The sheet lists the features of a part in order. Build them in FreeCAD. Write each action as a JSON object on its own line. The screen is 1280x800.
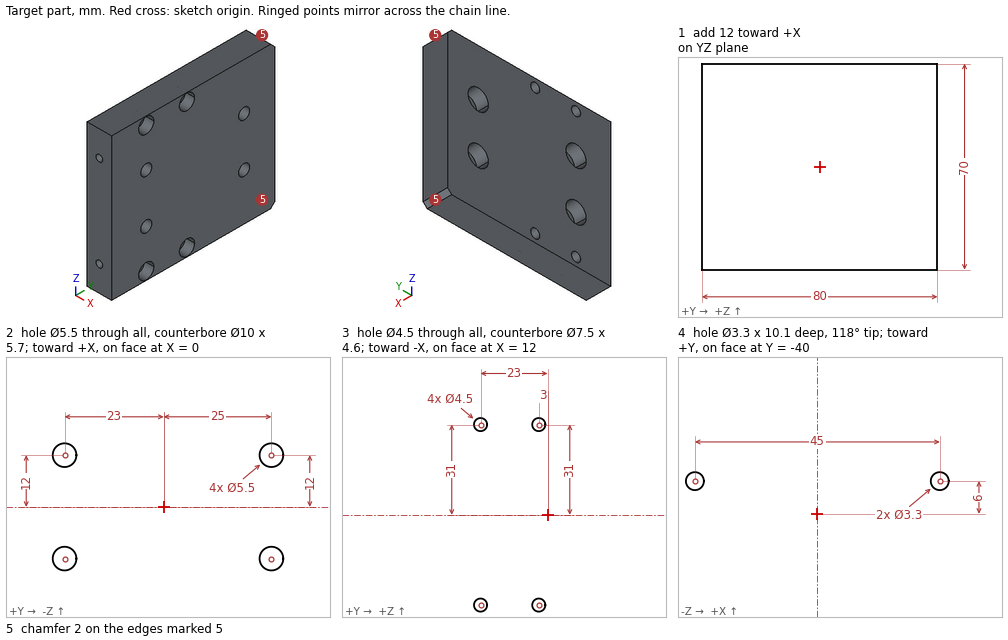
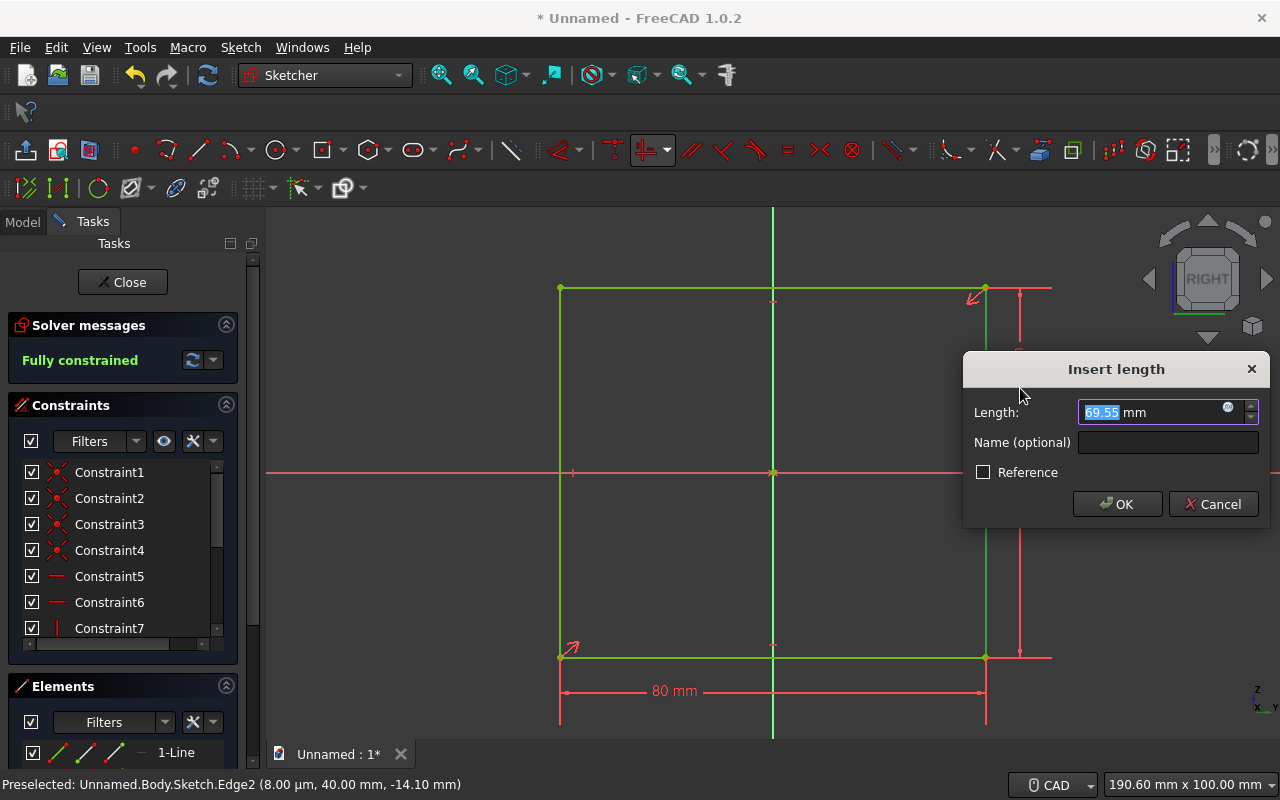
{"action": "type", "text": "70"}
{"action": "key", "text": "Return"}
{"action": "key", "text": "Escape"}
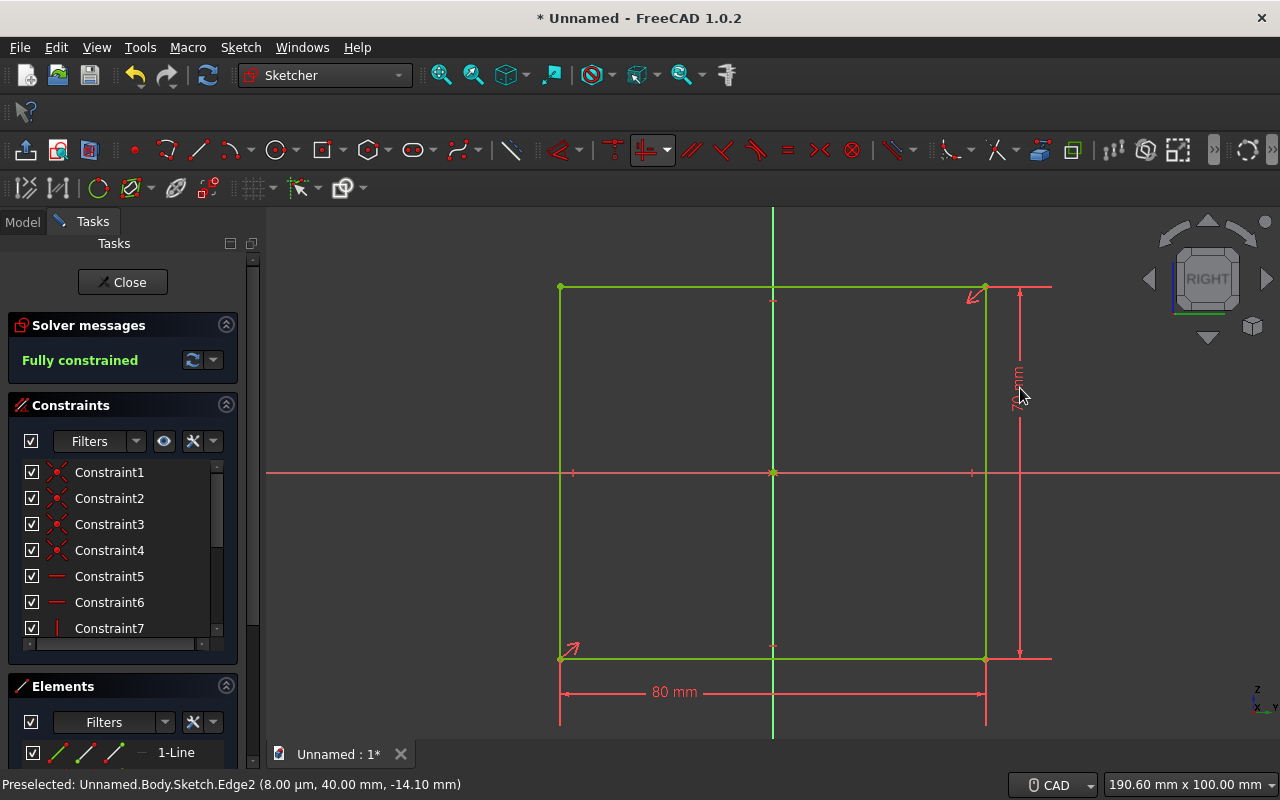
{"action": "left_click", "coordinate": [123, 282]}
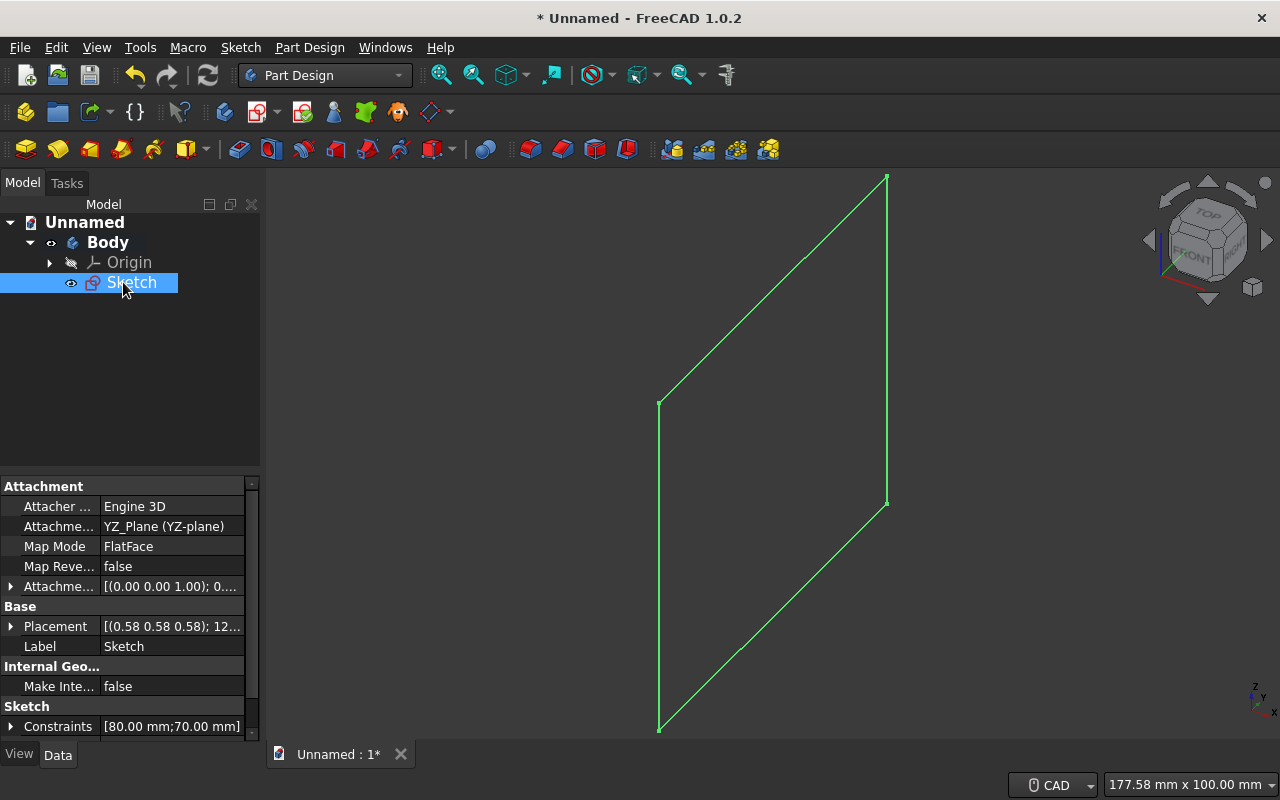
{"action": "left_click", "coordinate": [26, 150]}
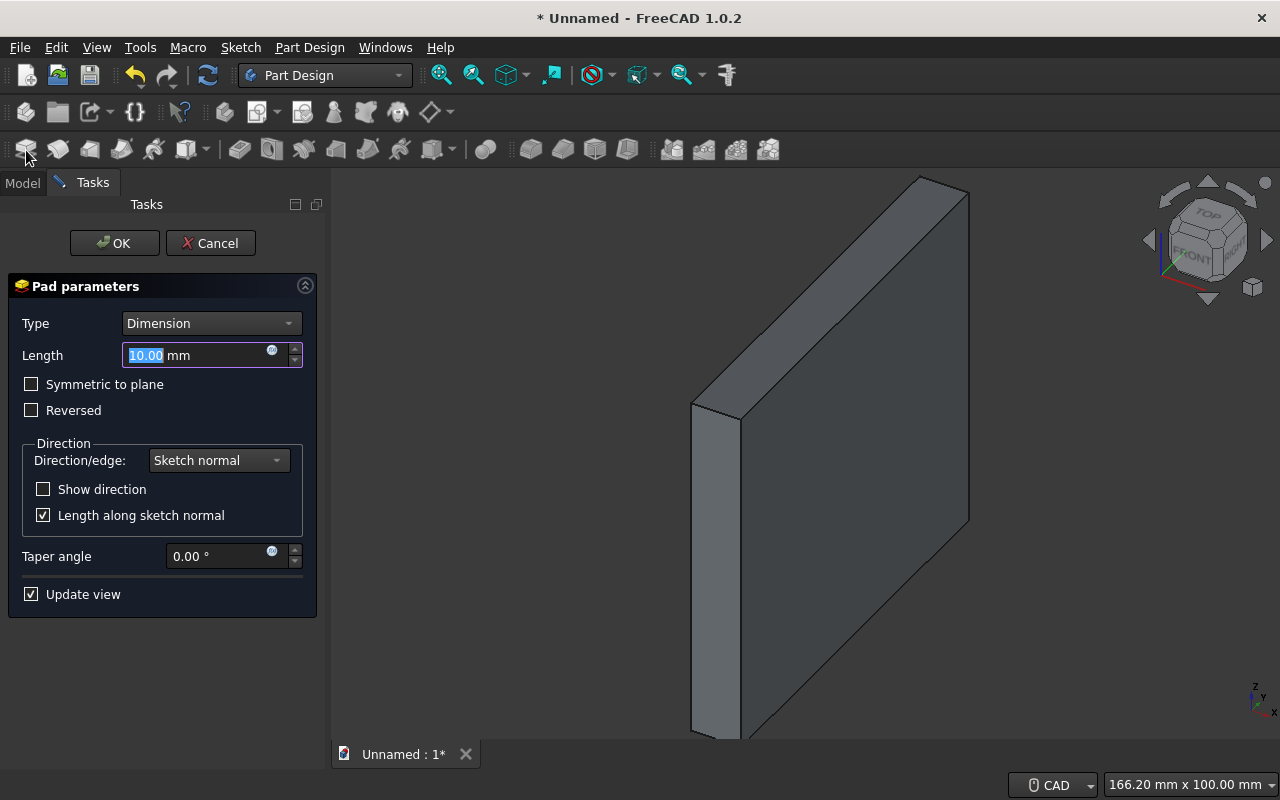
{"action": "type", "text": "12"}
{"action": "key", "text": "Tab"}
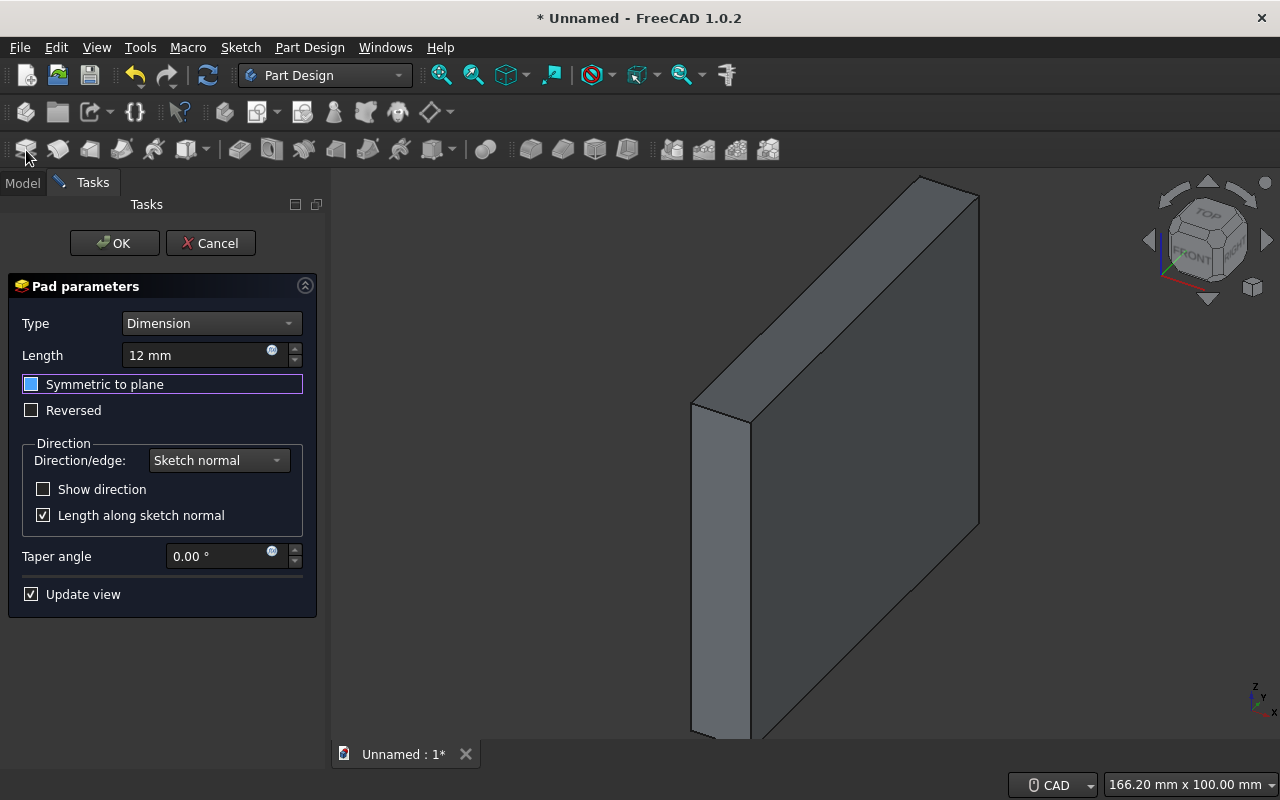
{"action": "left_click", "coordinate": [115, 243]}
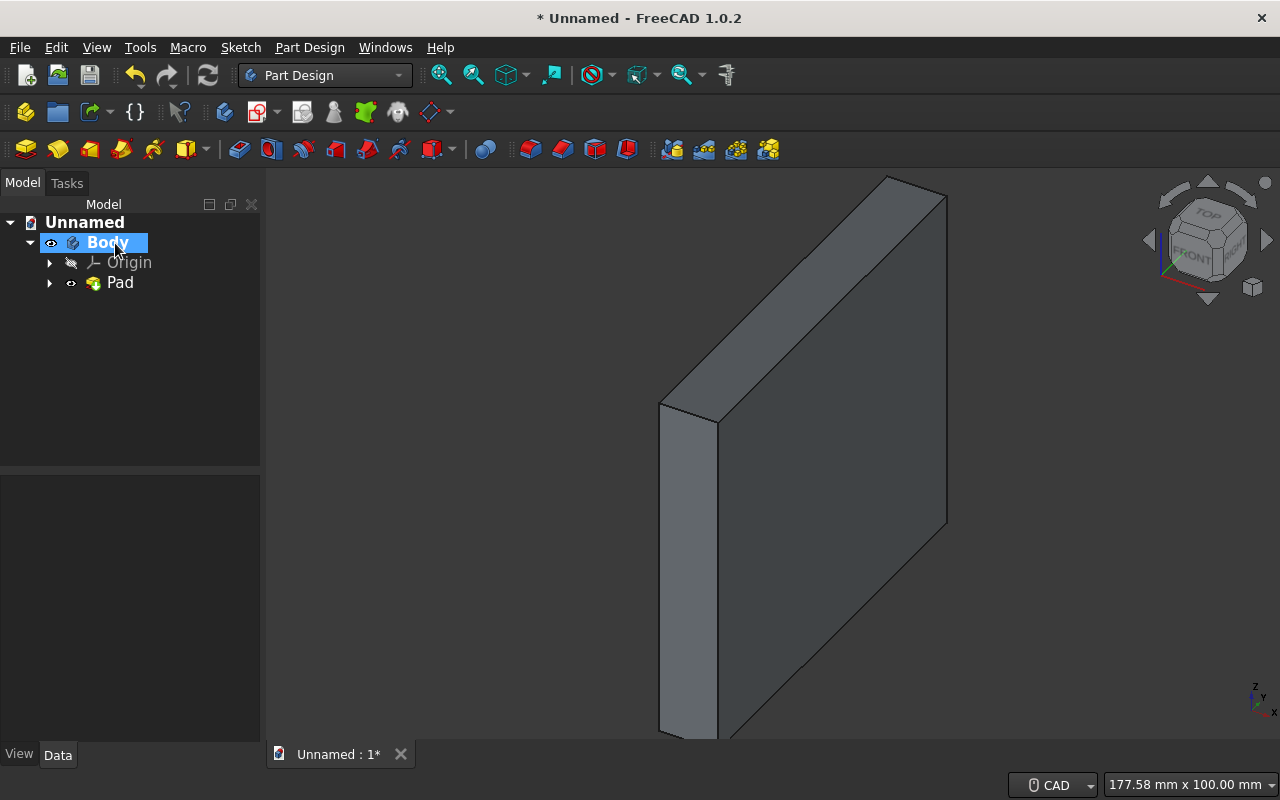
{"action": "left_click", "coordinate": [442, 76]}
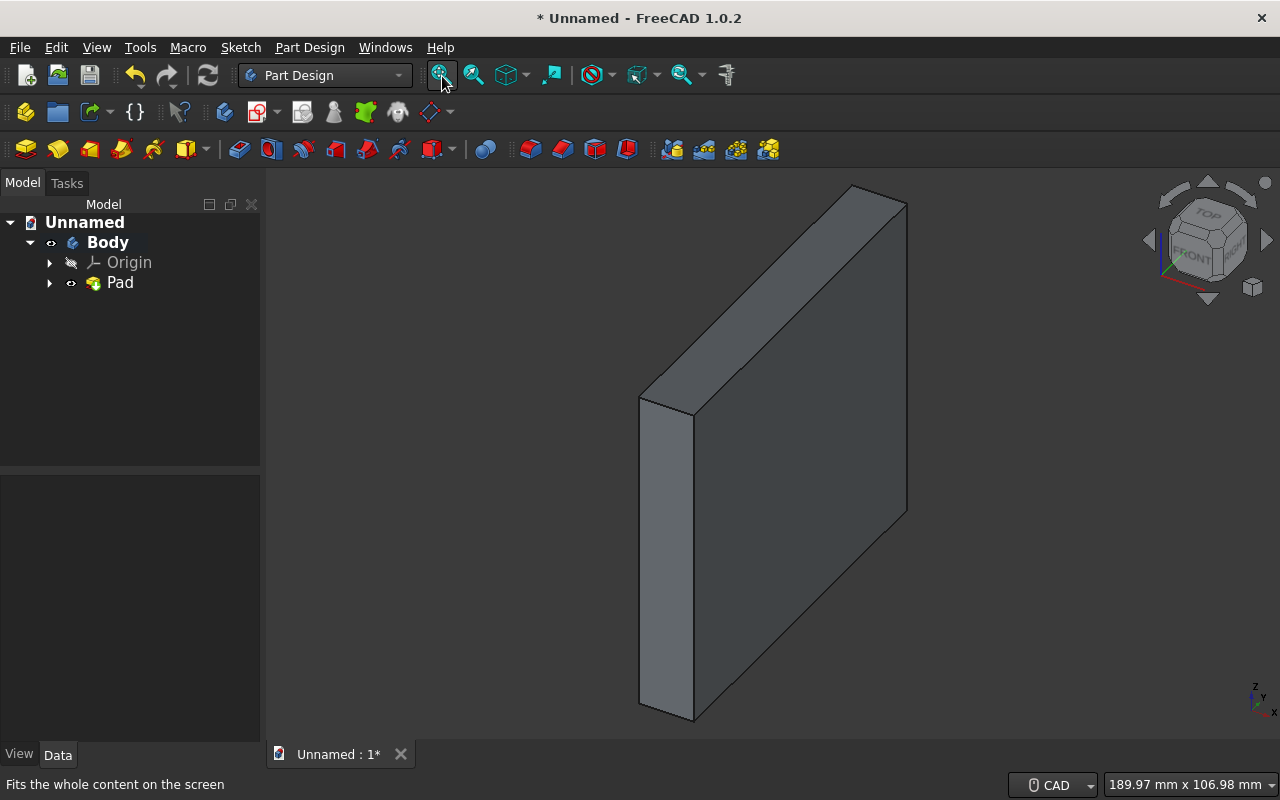
{"action": "key", "text": "6"}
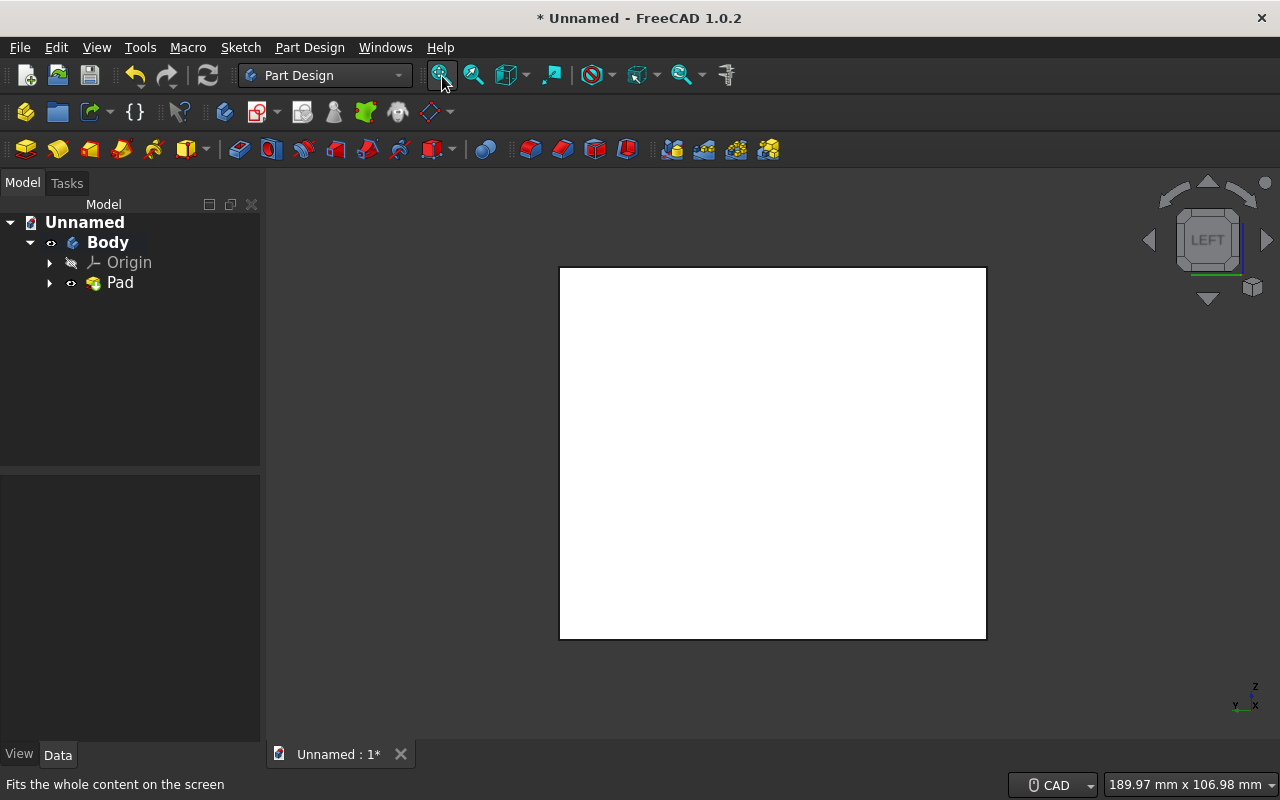
{"action": "left_click", "coordinate": [773, 452]}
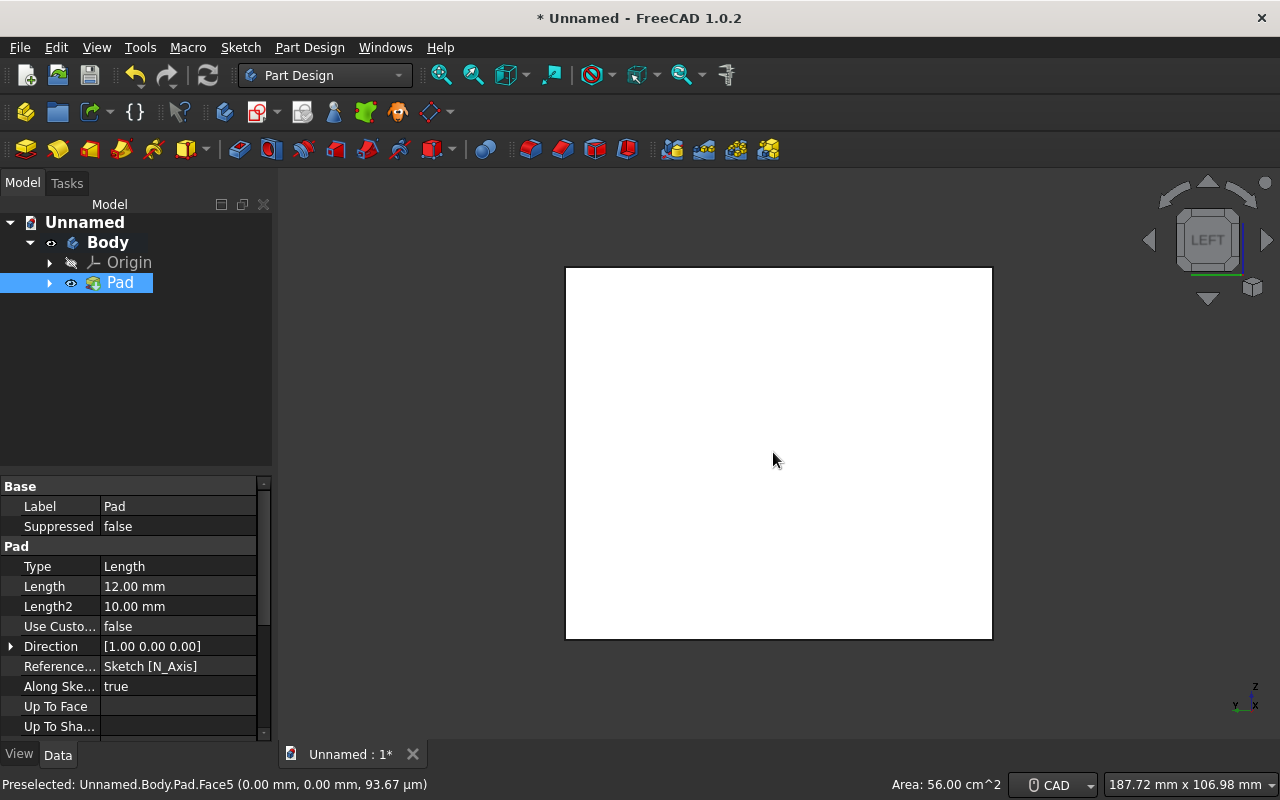
{"action": "left_click", "coordinate": [258, 112]}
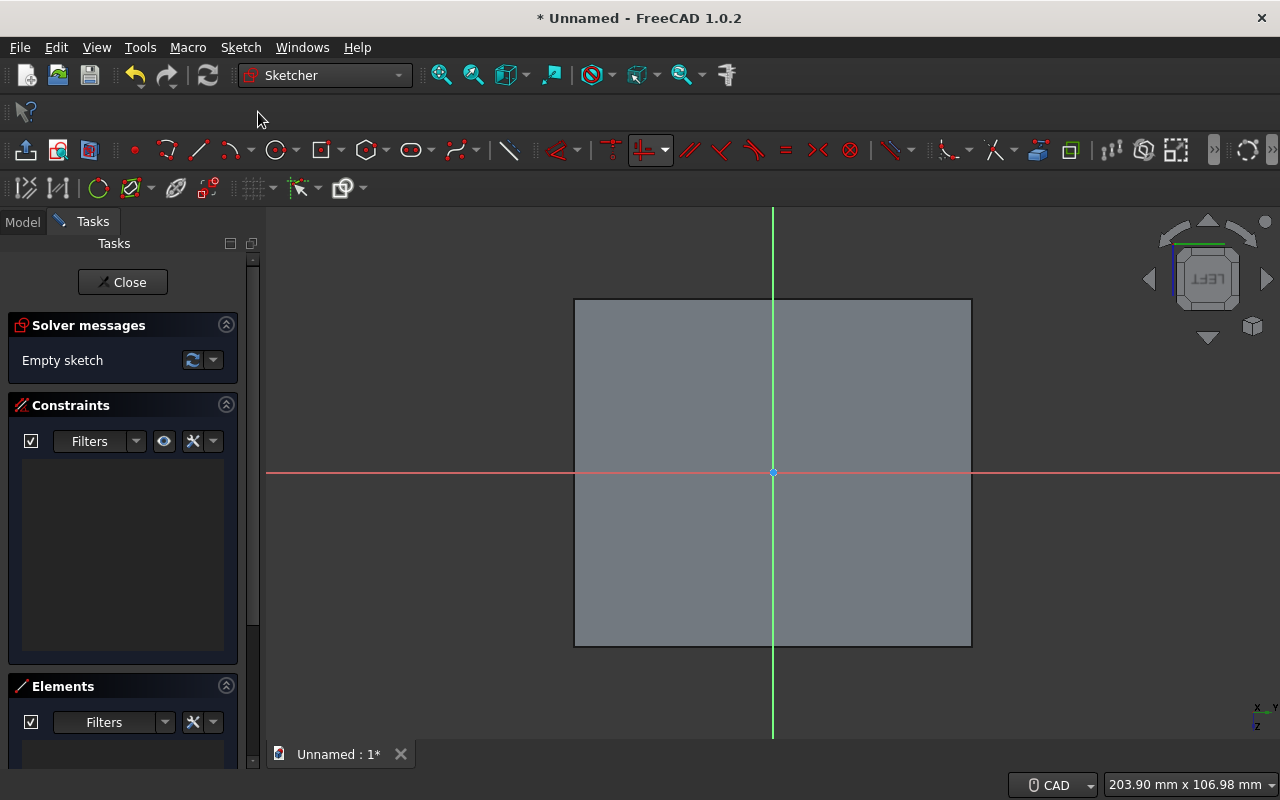
{"action": "scroll", "coordinate": [838, 473], "scroll_direction": "up", "scroll_amount": 4}